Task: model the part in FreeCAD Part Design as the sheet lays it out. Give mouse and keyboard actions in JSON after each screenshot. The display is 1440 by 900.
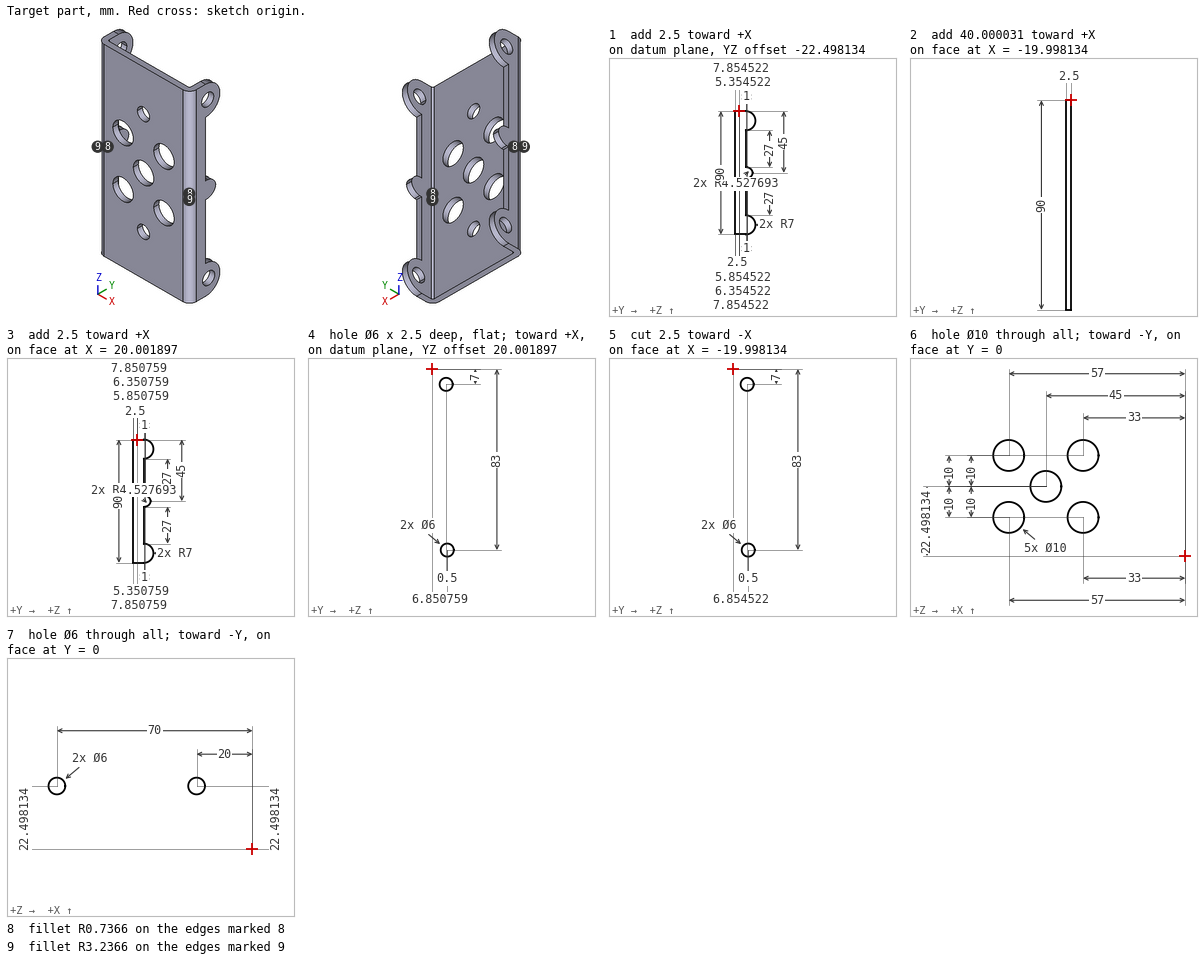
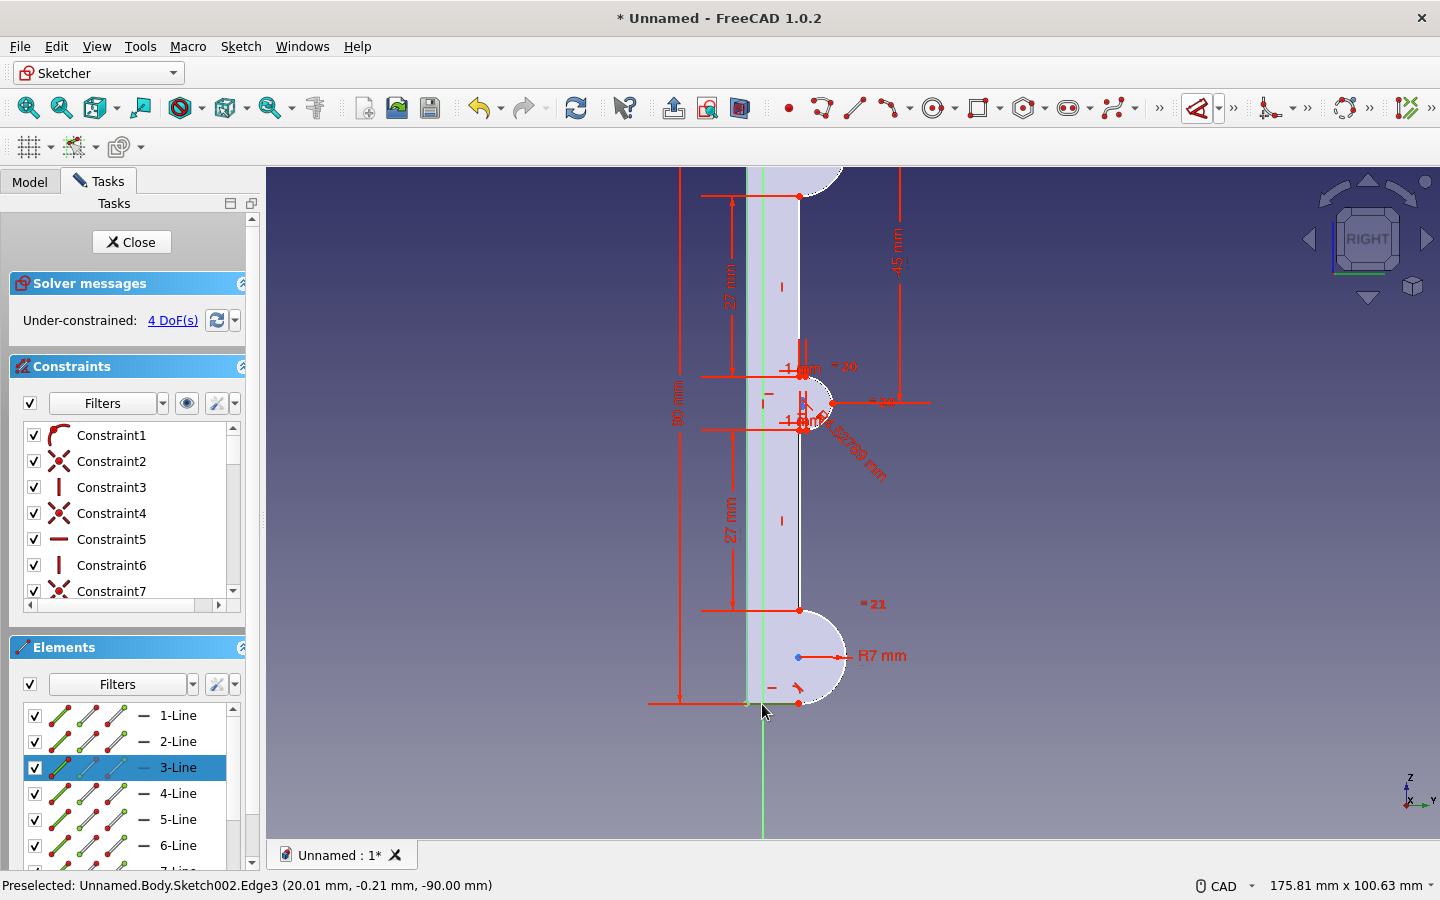
{"action": "key", "text": "l"}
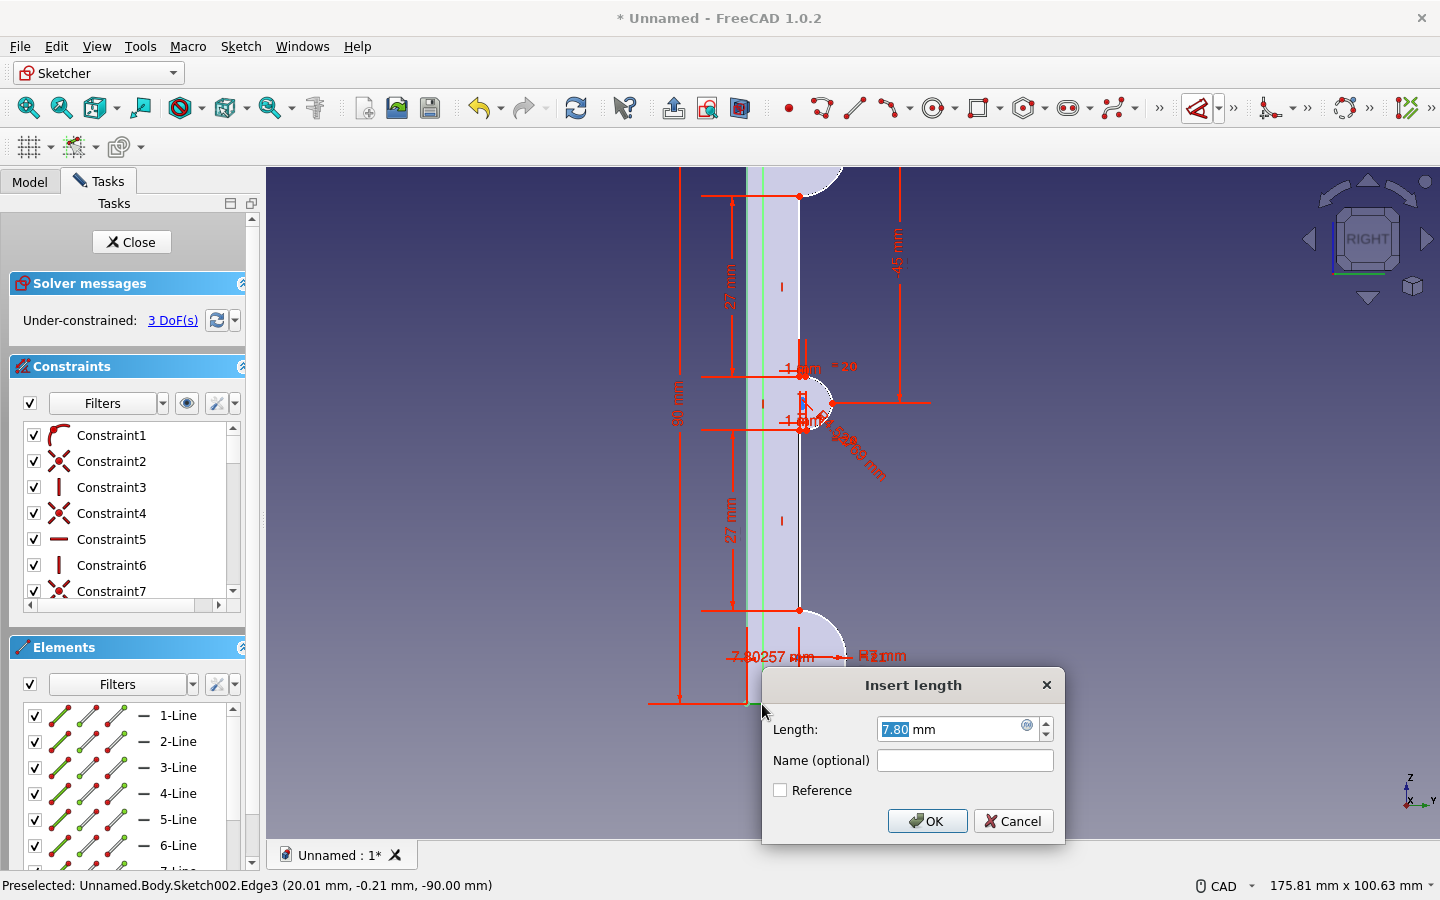
{"action": "type", "text": "7.850759"}
{"action": "key", "text": "Return"}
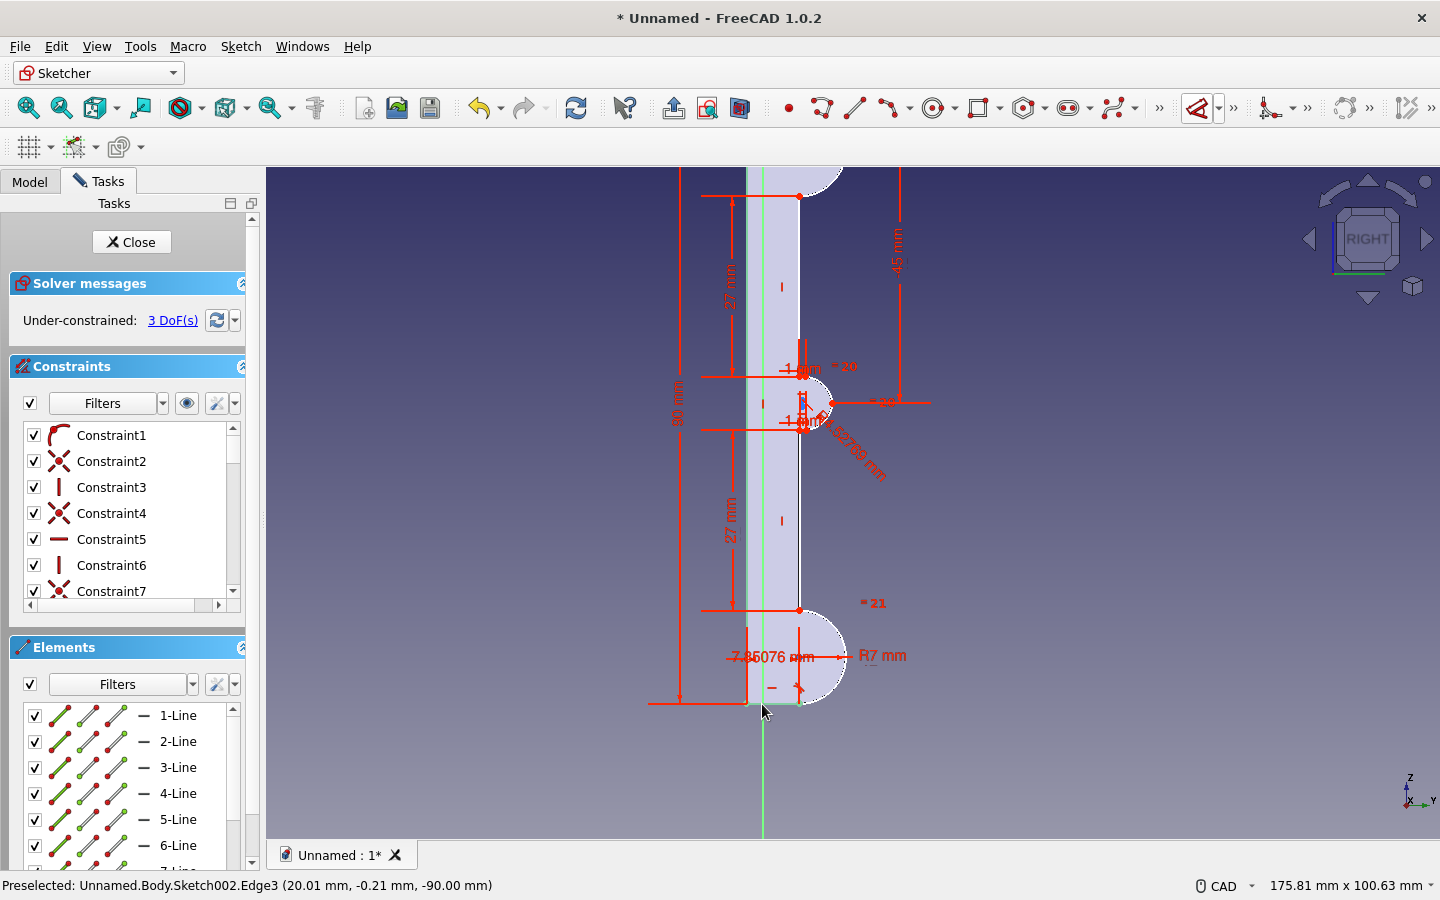
{"action": "left_click", "coordinate": [800, 611]}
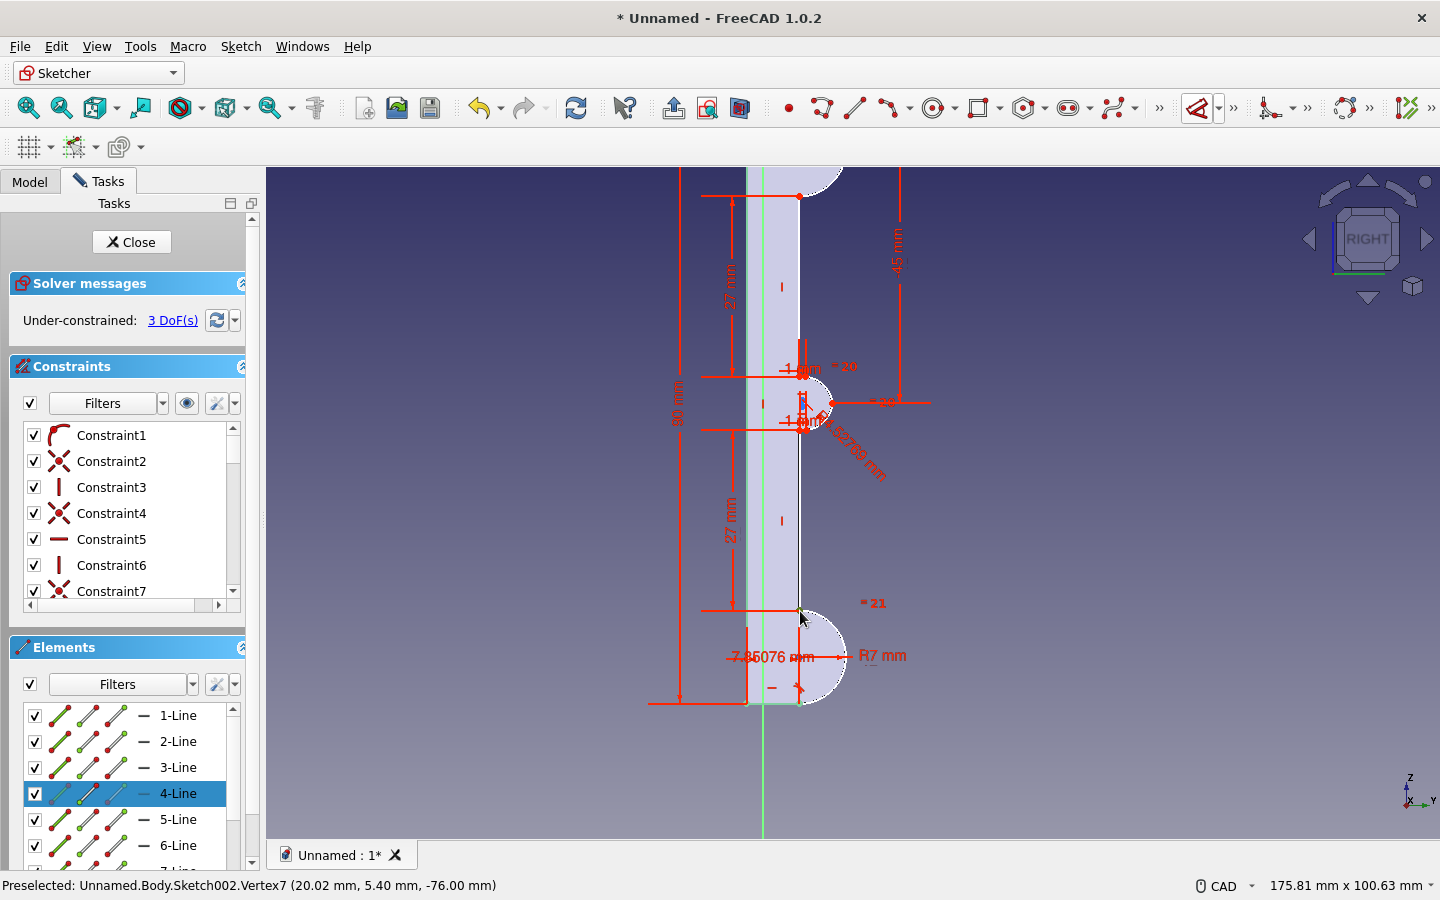
{"action": "key", "text": "l"}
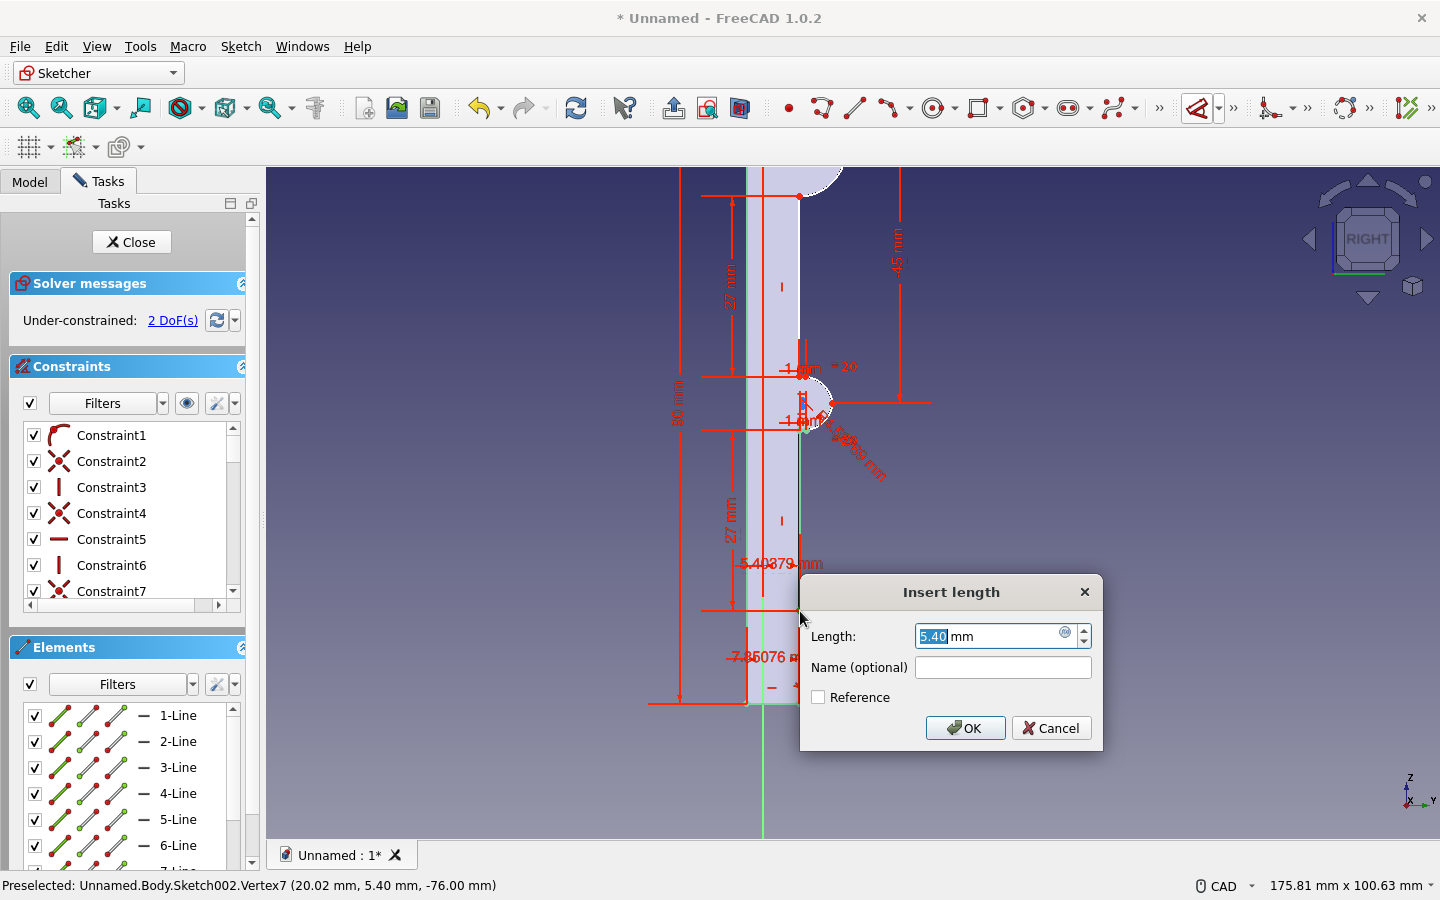
{"action": "type", "text": "5.350759"}
{"action": "key", "text": "Return"}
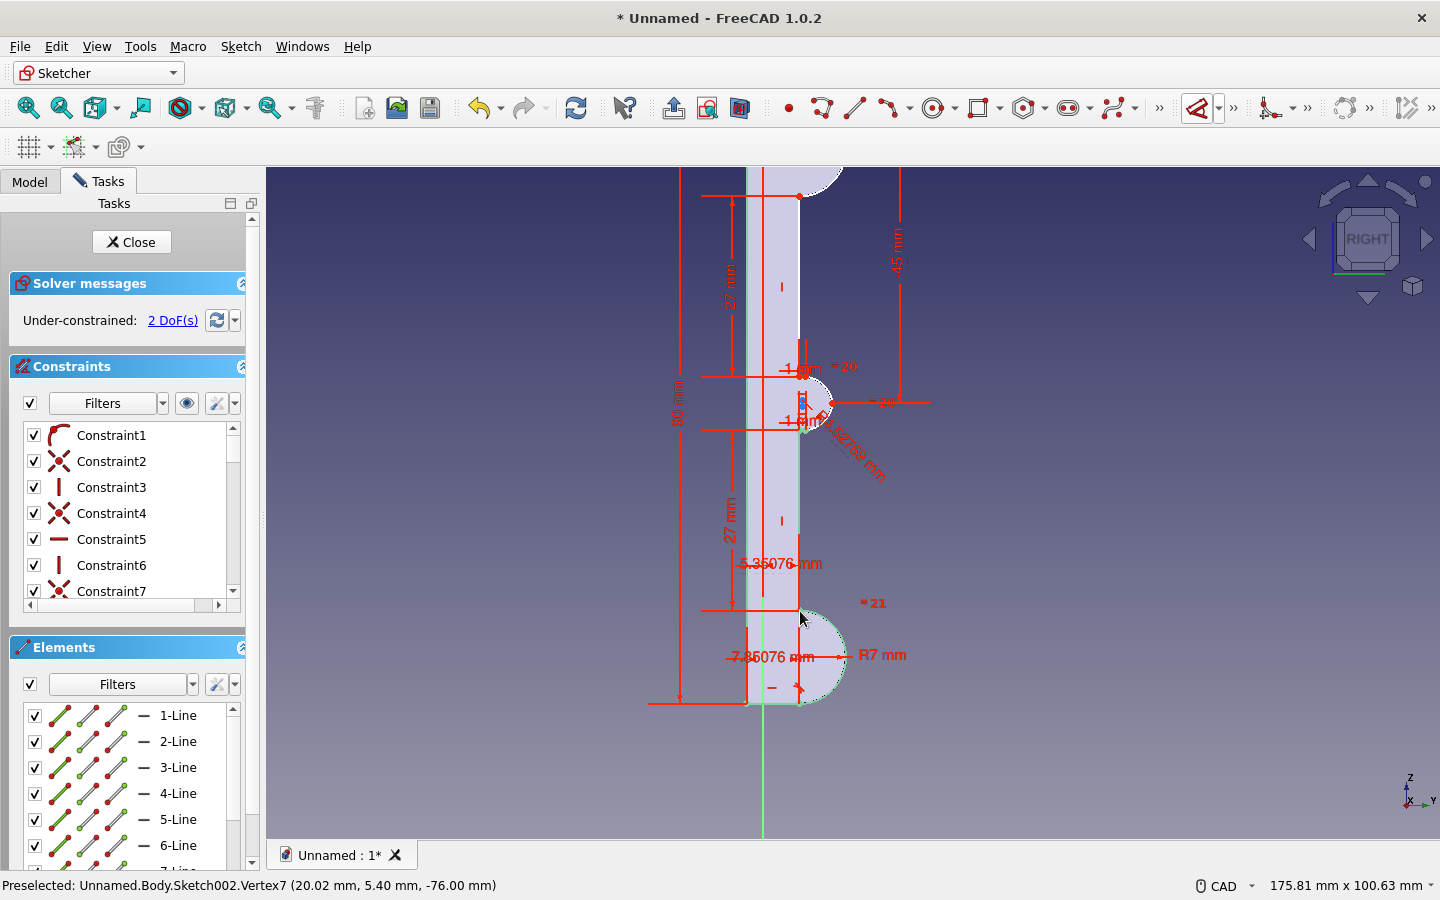
{"action": "scroll", "coordinate": [806, 377], "scroll_direction": "up", "scroll_amount": 4}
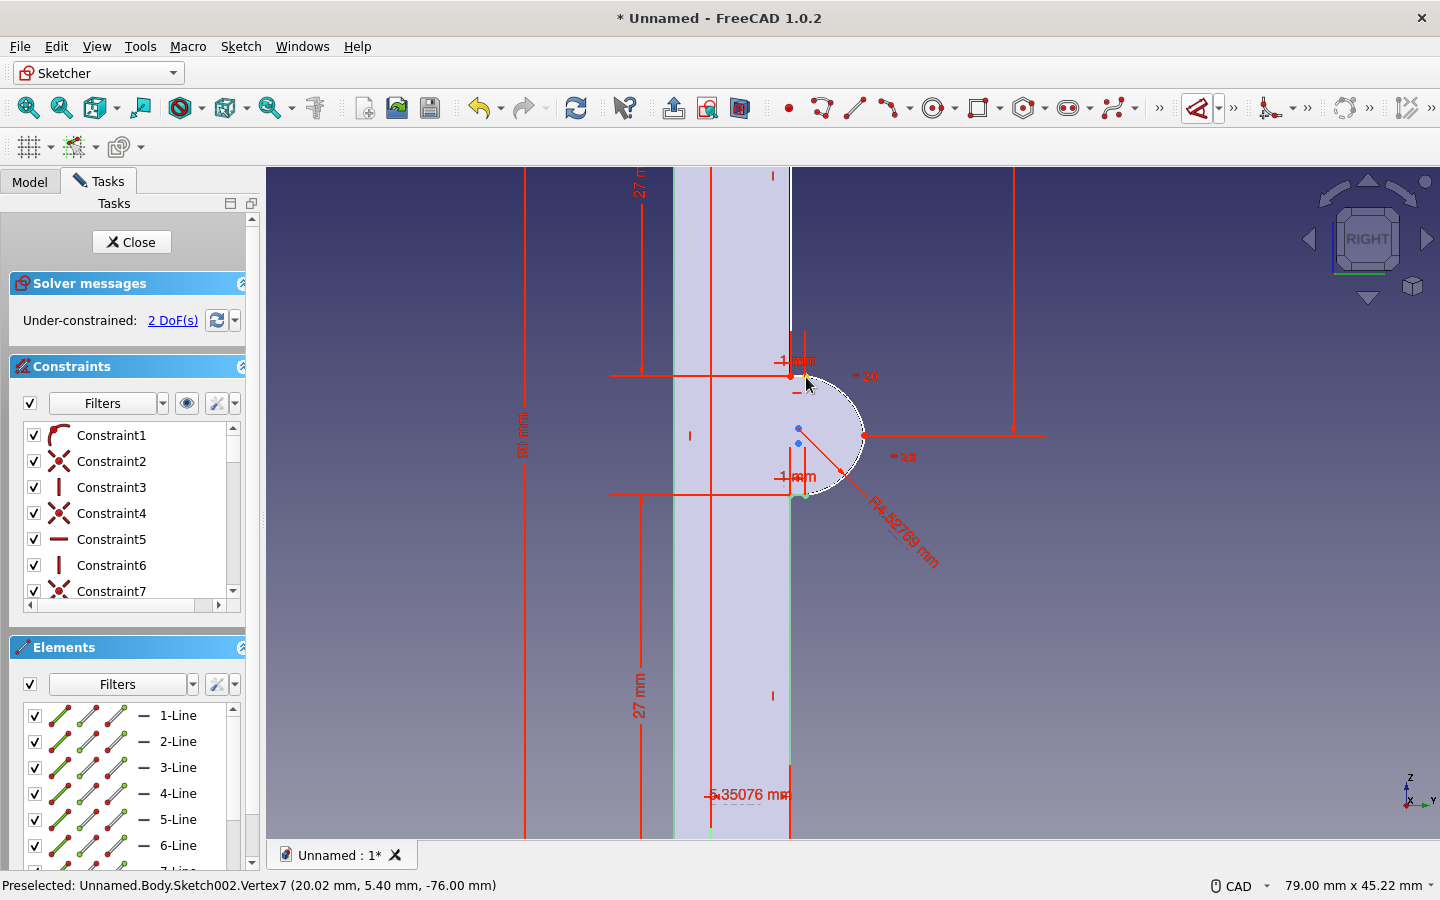
{"action": "left_click", "coordinate": [805, 376]}